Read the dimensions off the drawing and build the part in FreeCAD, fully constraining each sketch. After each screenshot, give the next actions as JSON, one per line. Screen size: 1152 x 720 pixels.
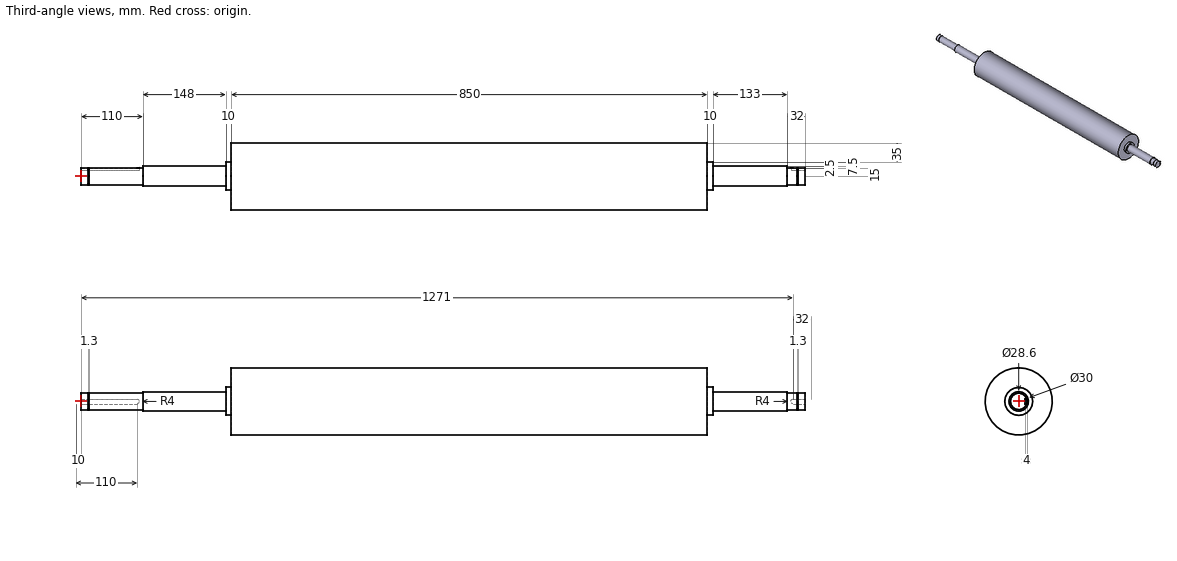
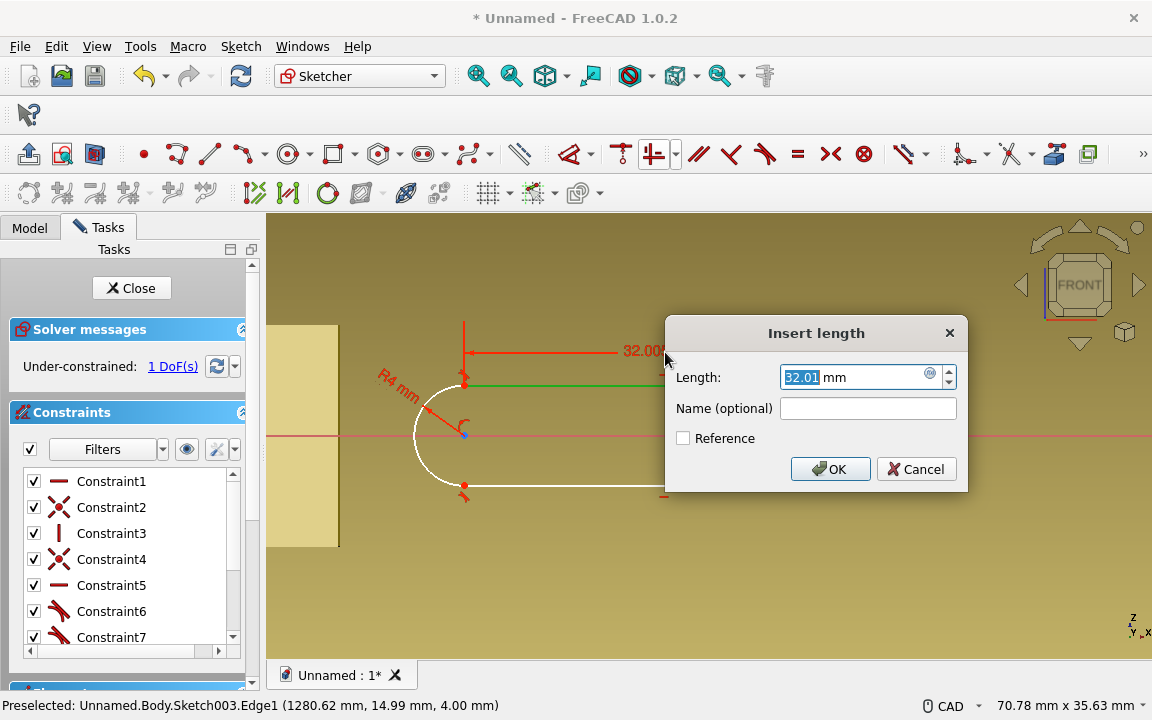
{"action": "type", "text": "32"}
{"action": "key", "text": "Return"}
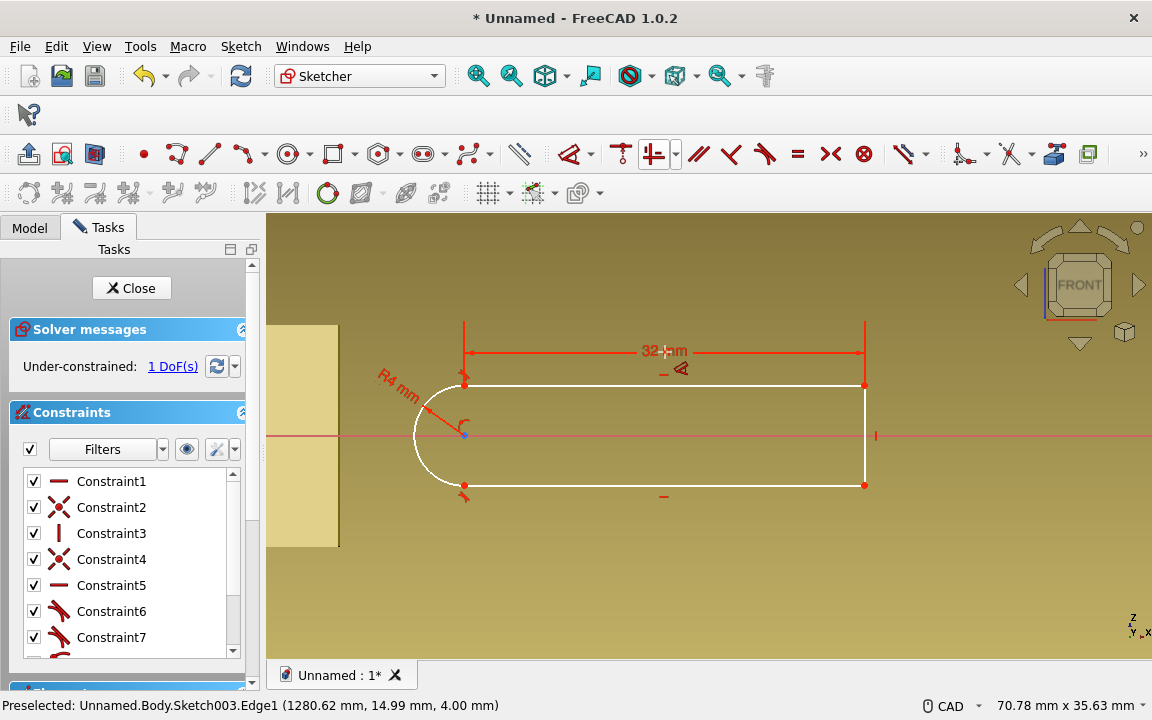
{"action": "left_click", "coordinate": [464, 386]}
{"action": "left_click", "coordinate": [379, 352]}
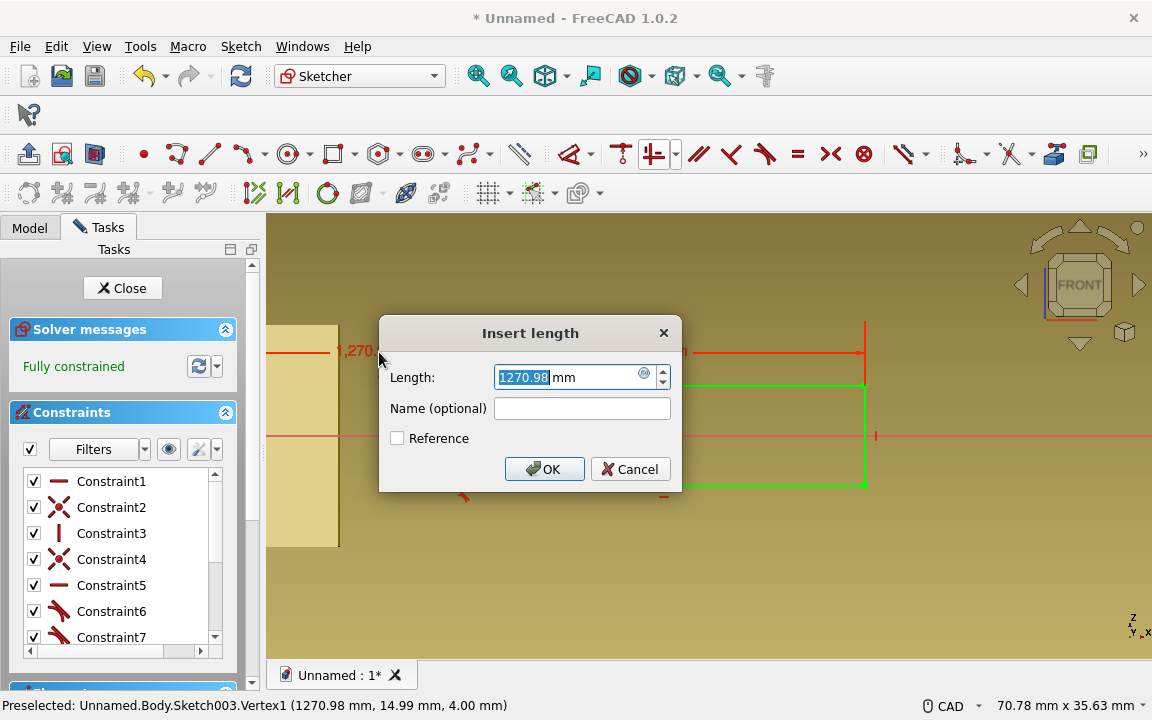
{"action": "type", "text": "1271"}
{"action": "key", "text": "Return"}
{"action": "key", "text": "Escape"}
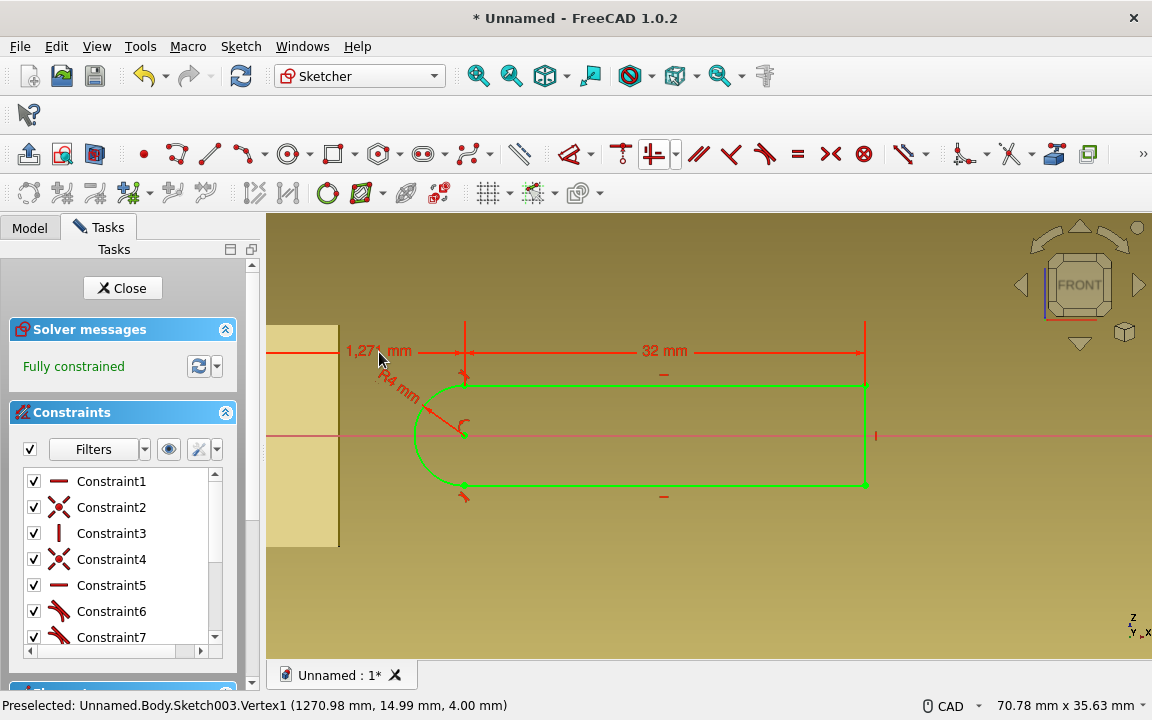
{"action": "left_click", "coordinate": [123, 288]}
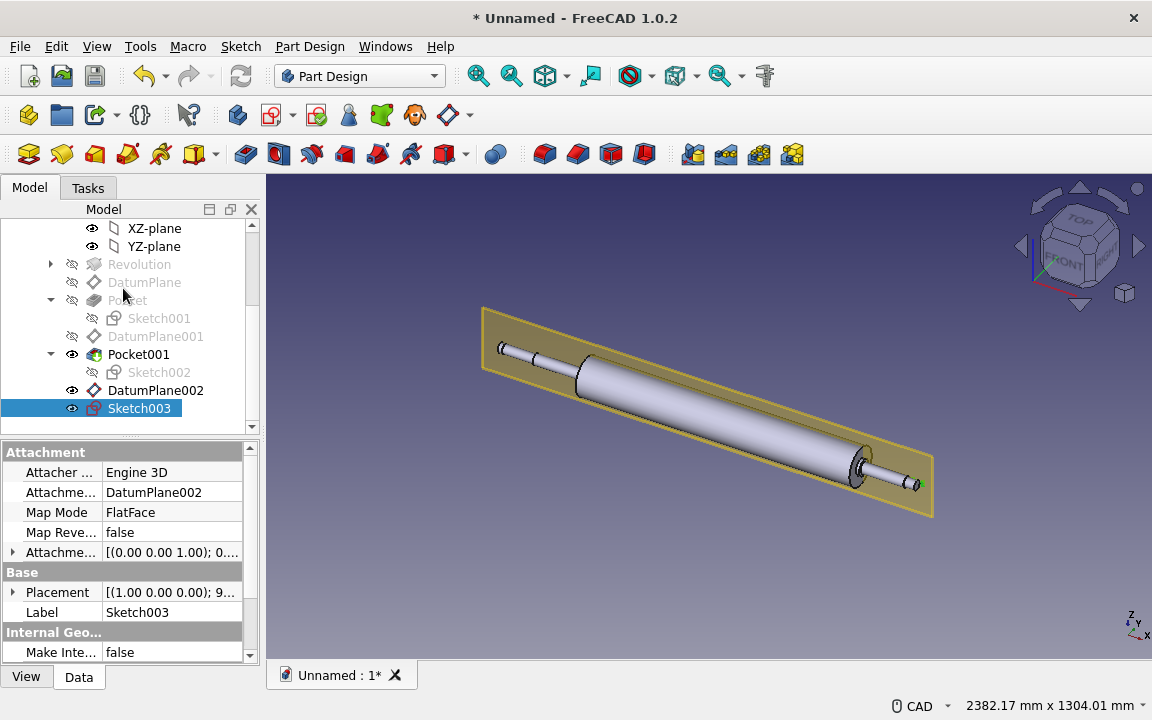
{"action": "left_click", "coordinate": [246, 154]}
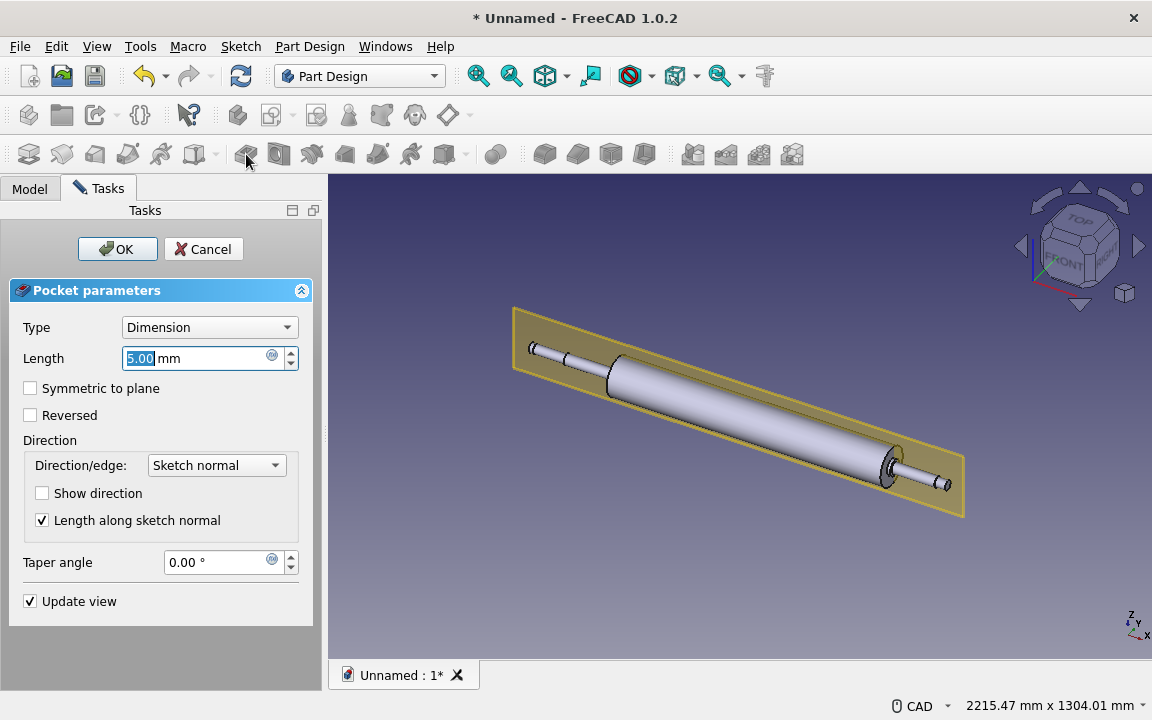
{"action": "type", "text": "4"}
{"action": "key", "text": "Tab"}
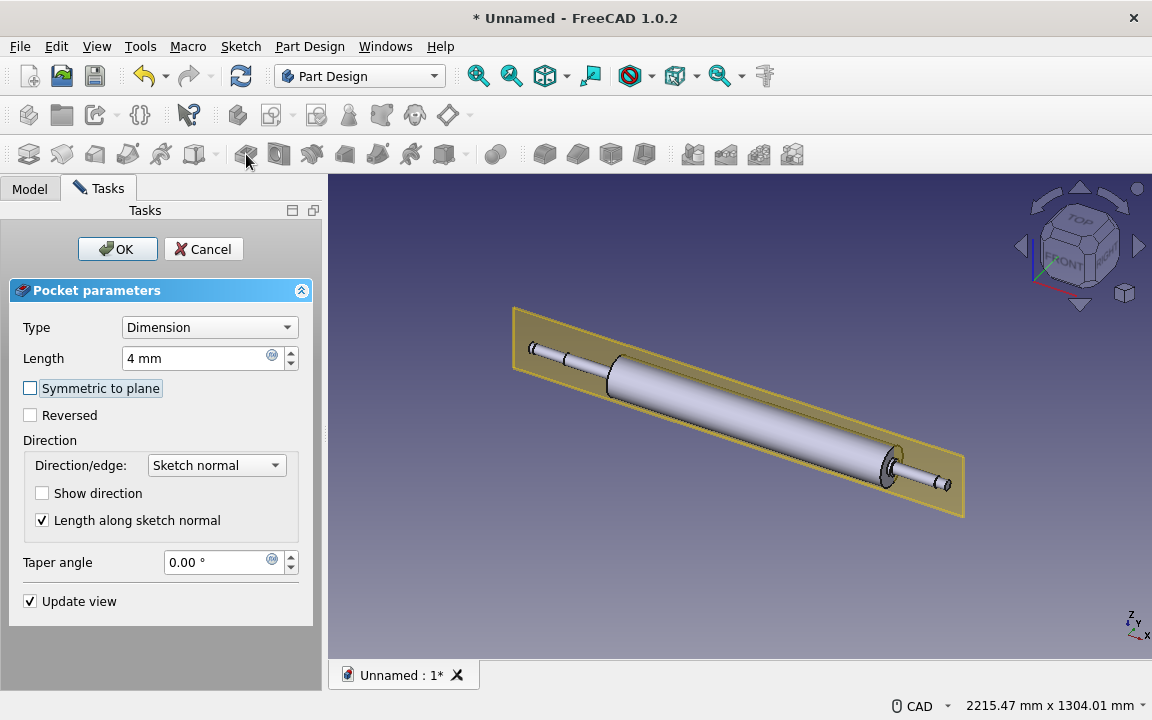
{"action": "left_click", "coordinate": [31, 415]}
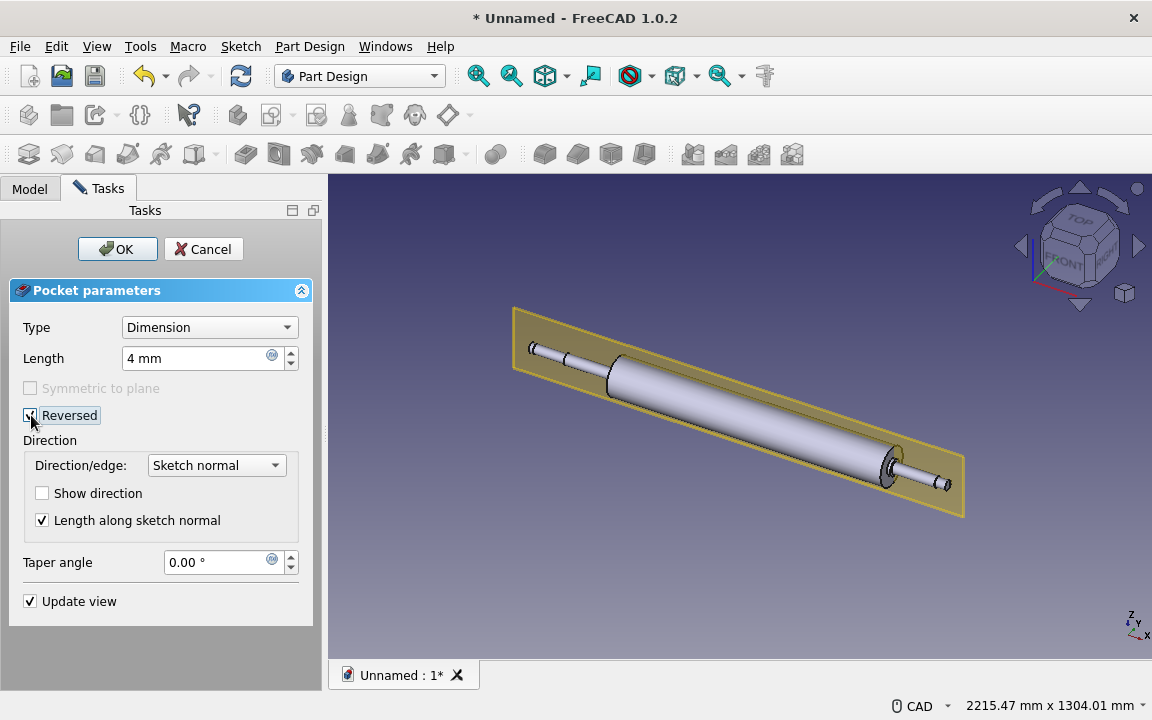
{"action": "left_click", "coordinate": [118, 249]}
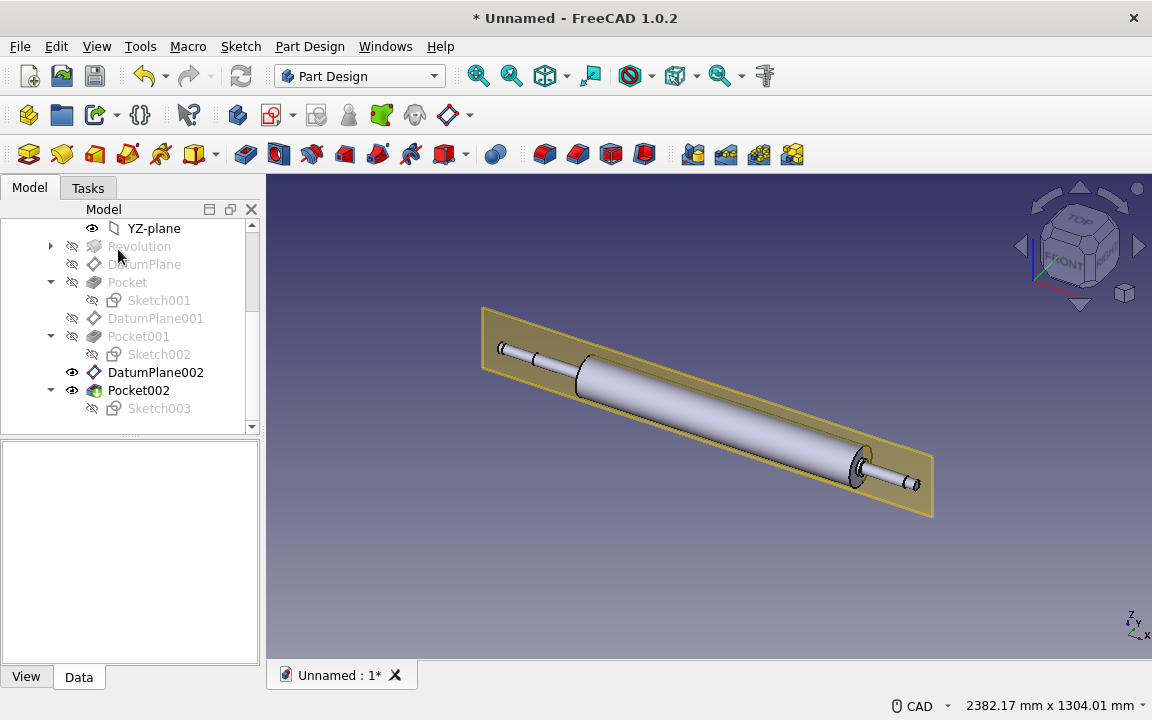
{"action": "left_click", "coordinate": [117, 372]}
{"action": "key", "text": "space"}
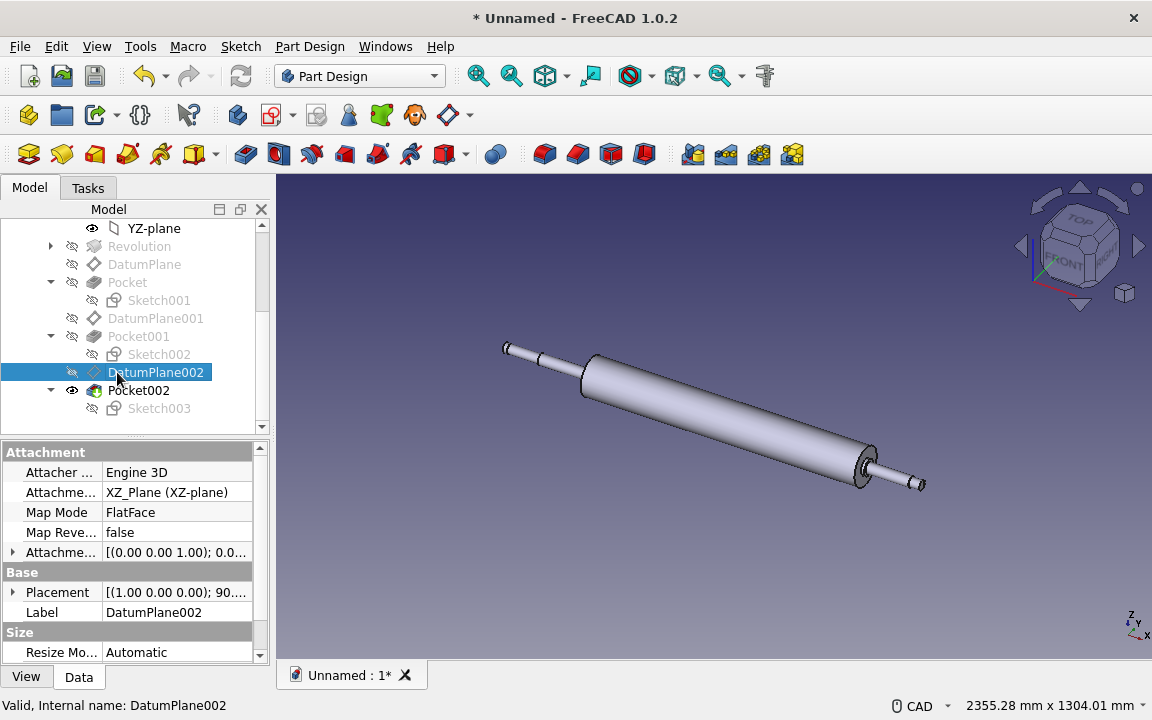
{"action": "scroll", "coordinate": [161, 314], "scroll_direction": "down", "scroll_amount": 3}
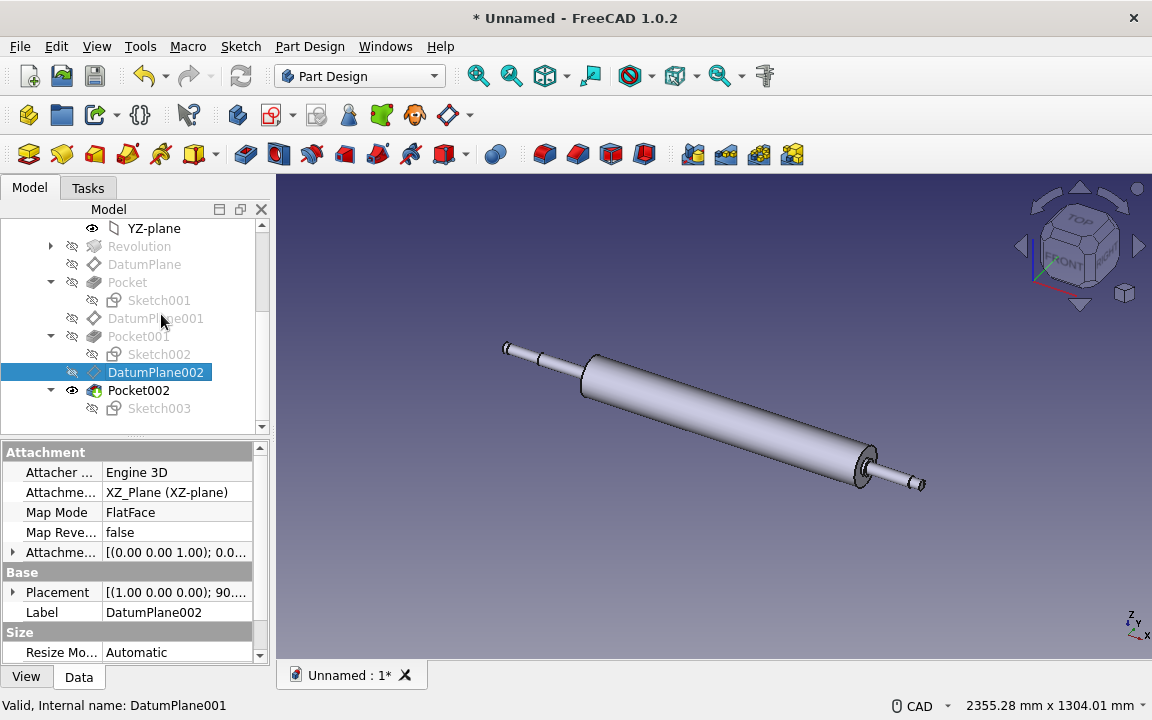
{"action": "scroll", "coordinate": [161, 314], "scroll_direction": "up", "scroll_amount": 15}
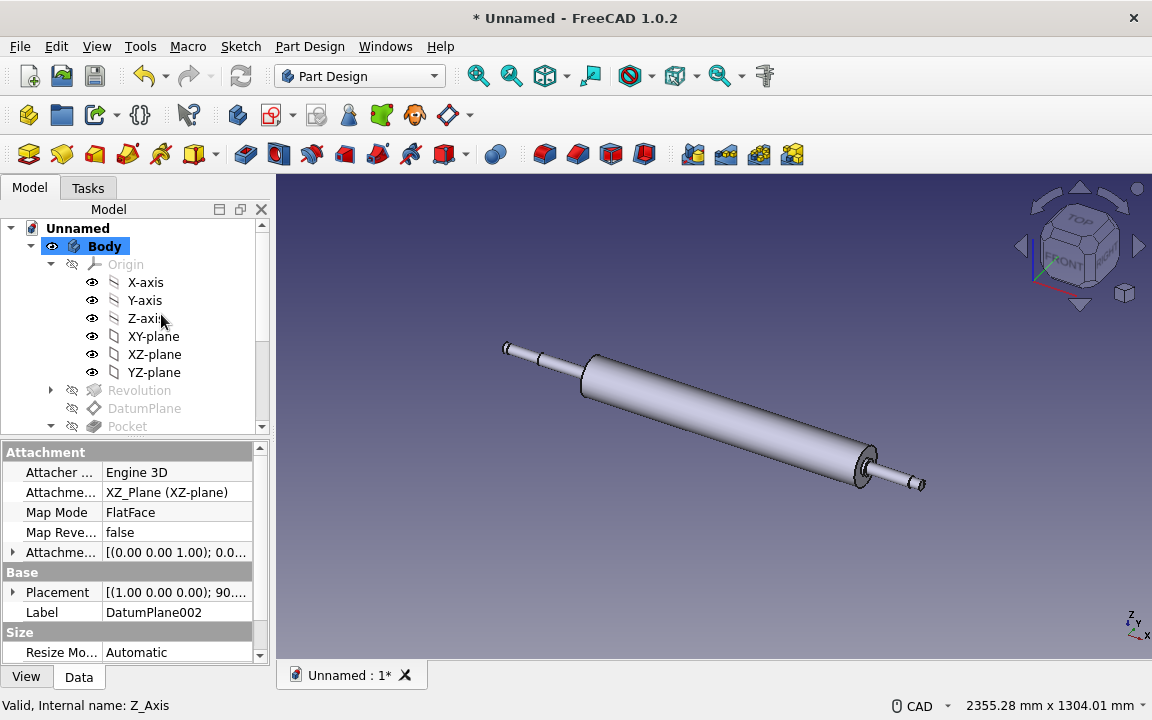
{"action": "left_click", "coordinate": [137, 372]}